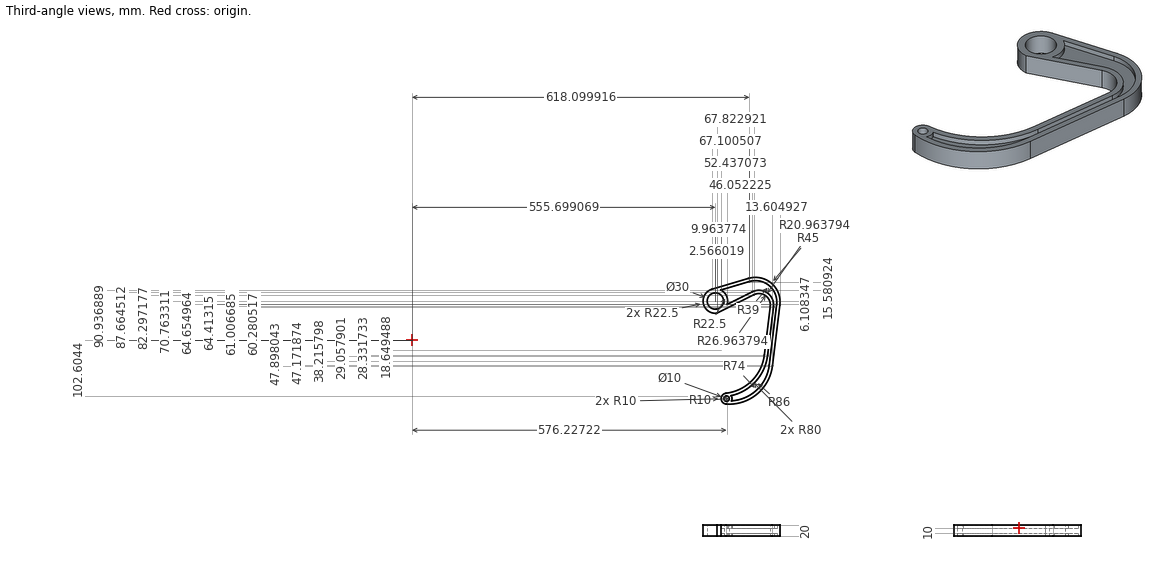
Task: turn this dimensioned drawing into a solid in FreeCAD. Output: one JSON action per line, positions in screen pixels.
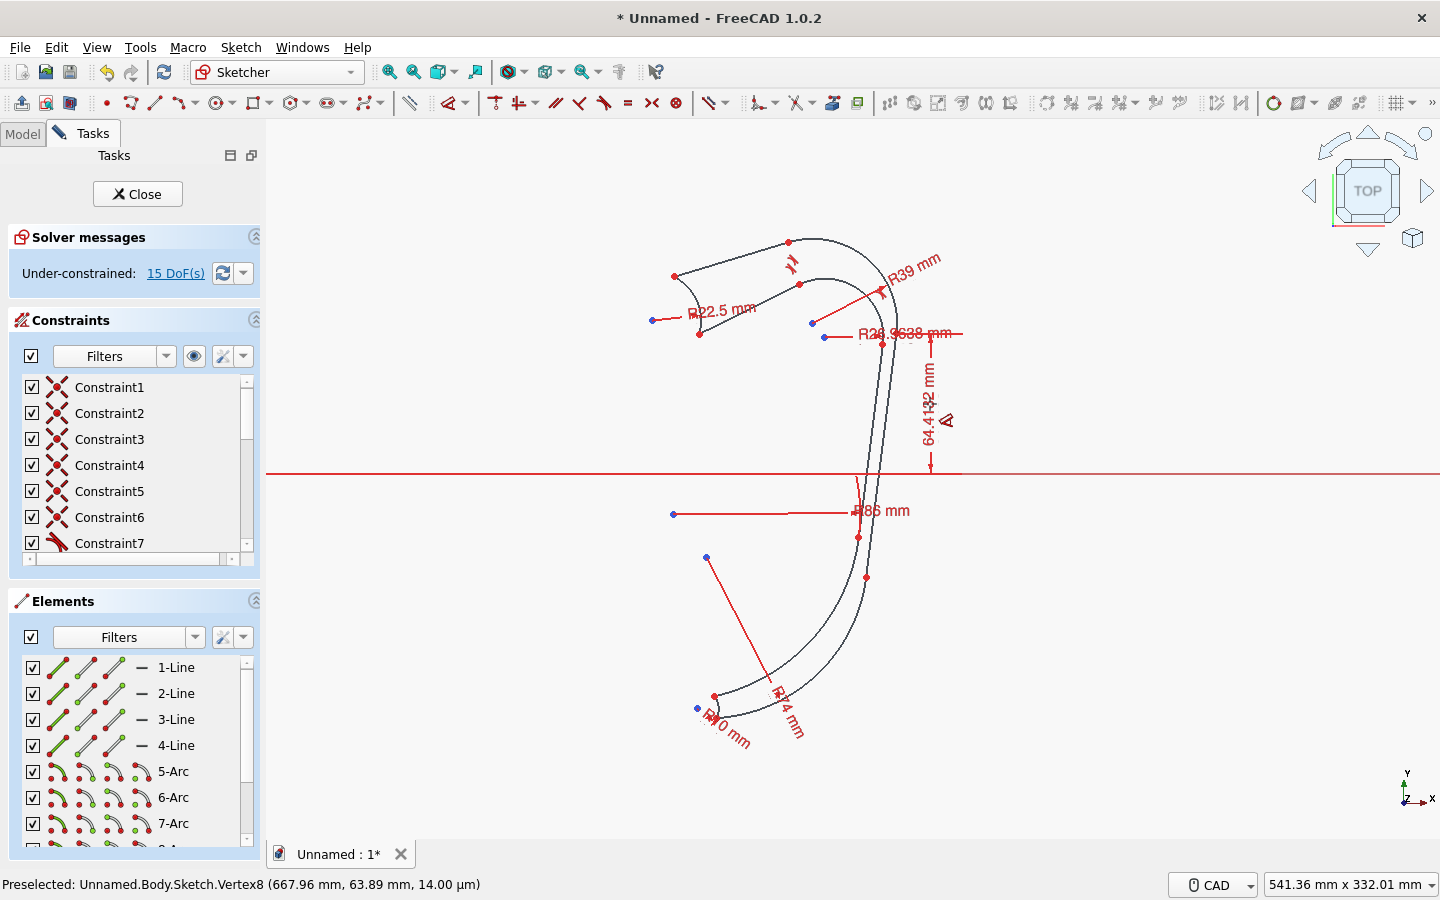
{"action": "left_click", "coordinate": [715, 696]}
{"action": "left_click", "coordinate": [749, 585]}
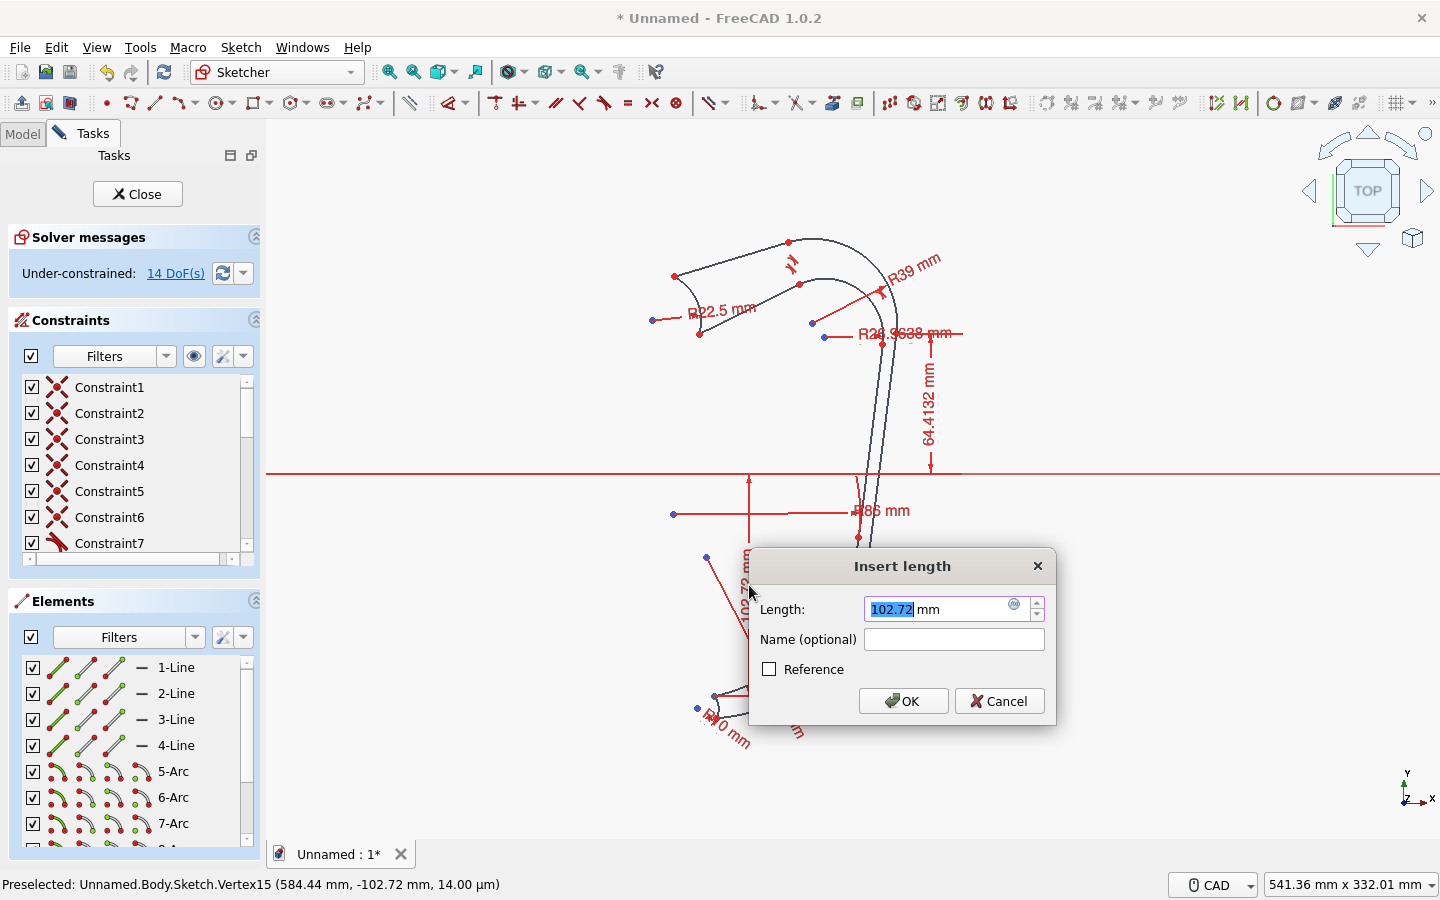
{"action": "type", "text": "102.6044"}
{"action": "key", "text": "Return"}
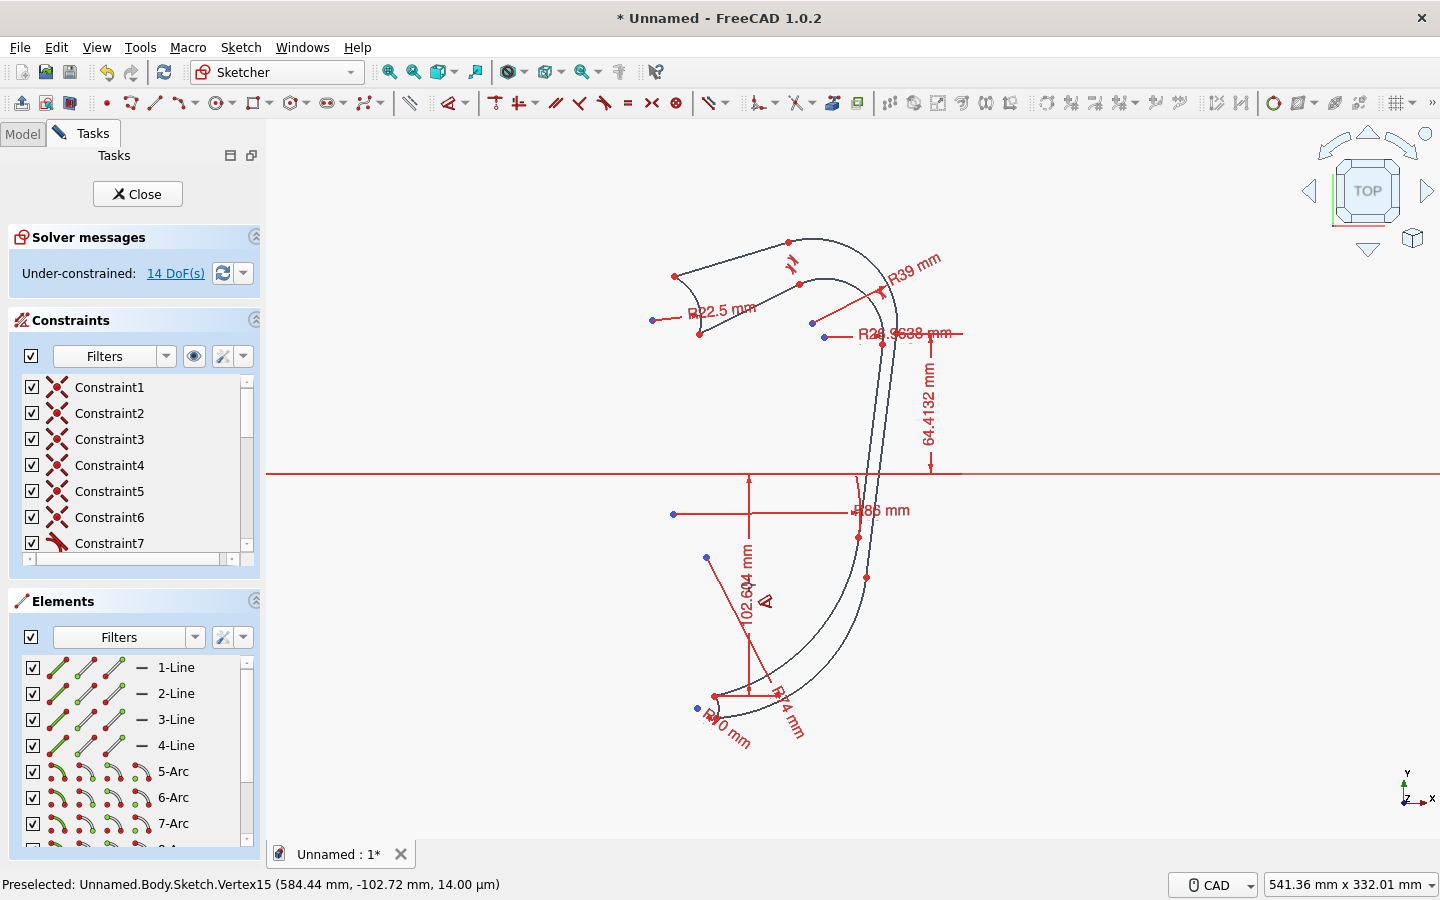
{"action": "left_click", "coordinate": [674, 277]}
{"action": "left_click", "coordinate": [708, 375]}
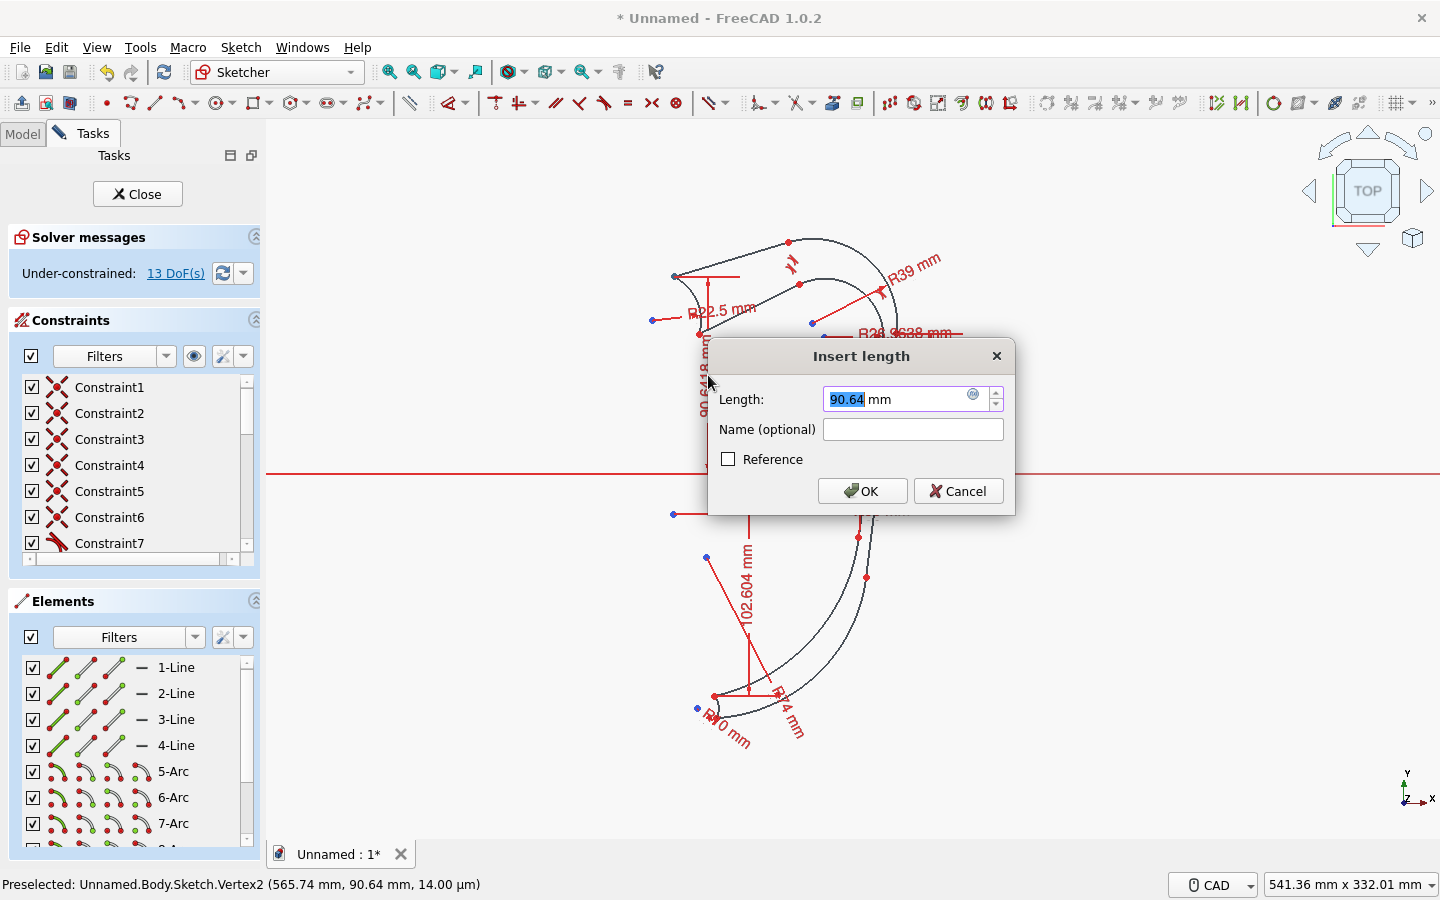
{"action": "type", "text": "90.936889"}
{"action": "key", "text": "Return"}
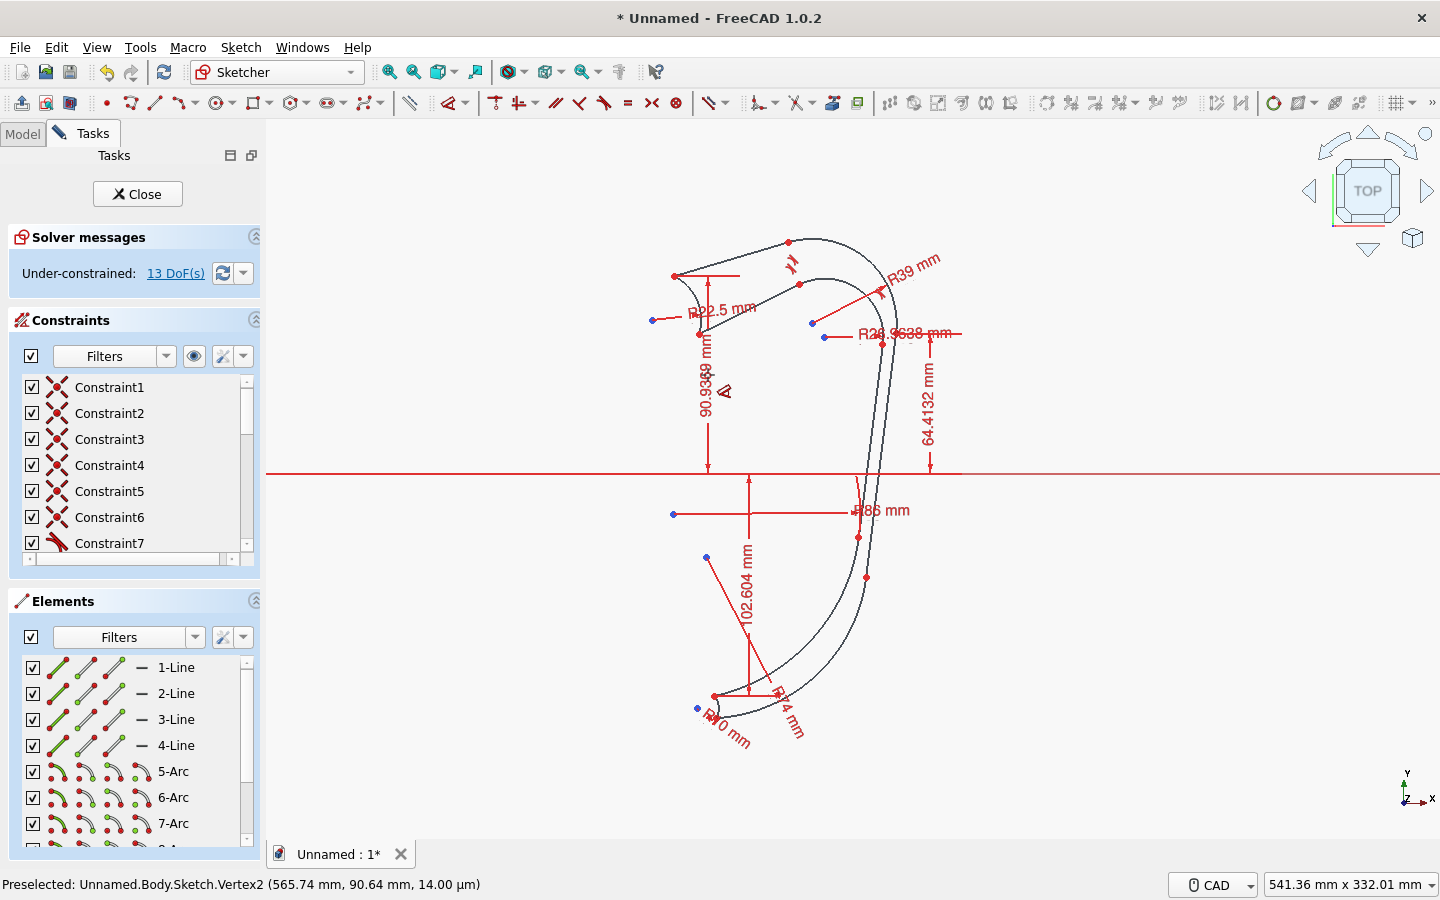
{"action": "left_click", "coordinate": [699, 334]}
{"action": "left_click", "coordinate": [733, 404]}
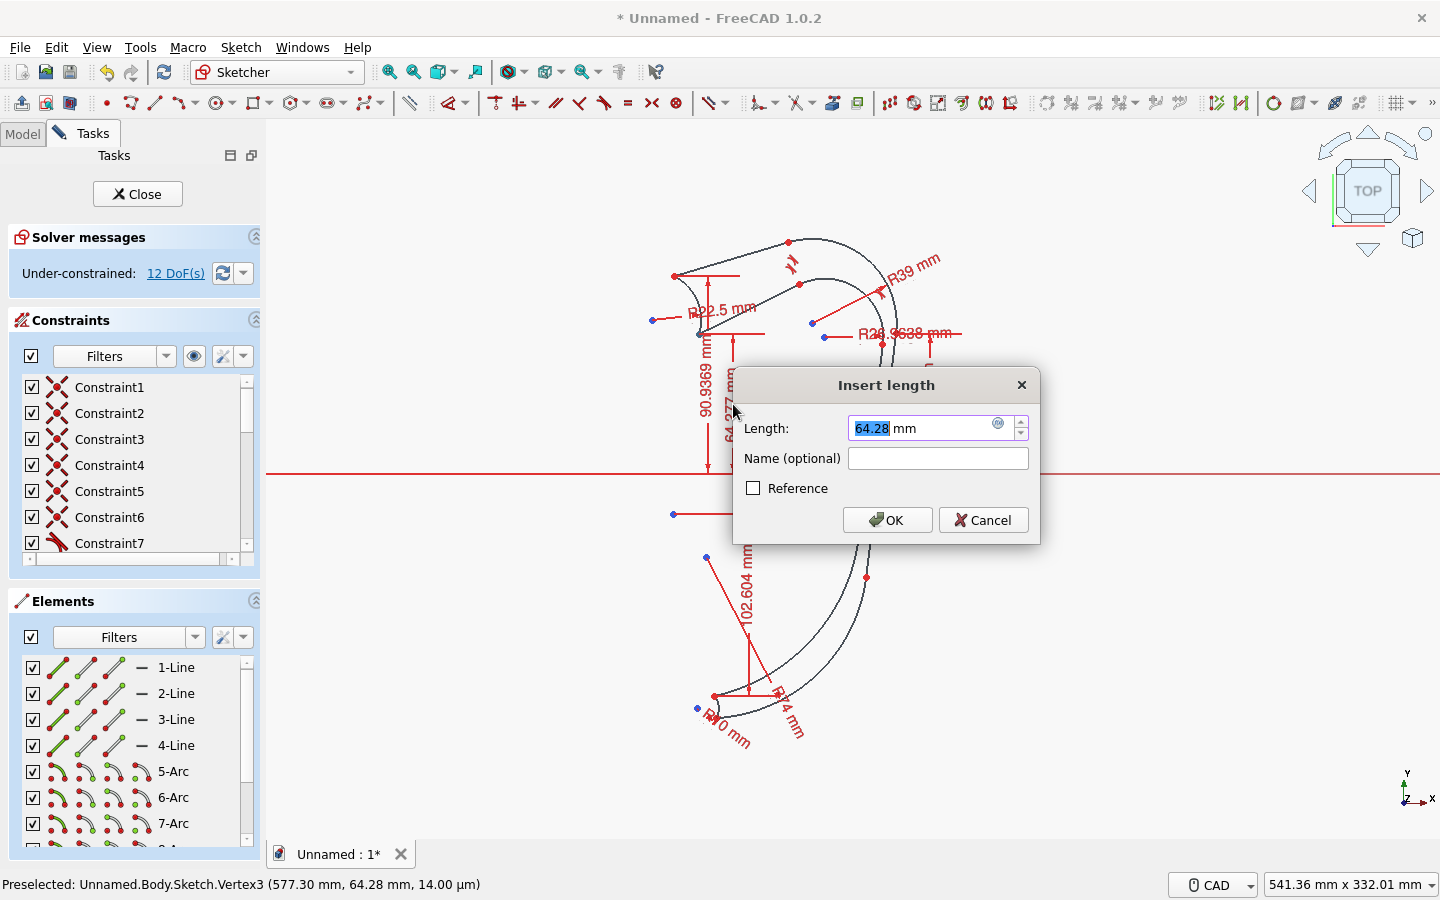
{"action": "type", "text": "64.654964"}
{"action": "key", "text": "Return"}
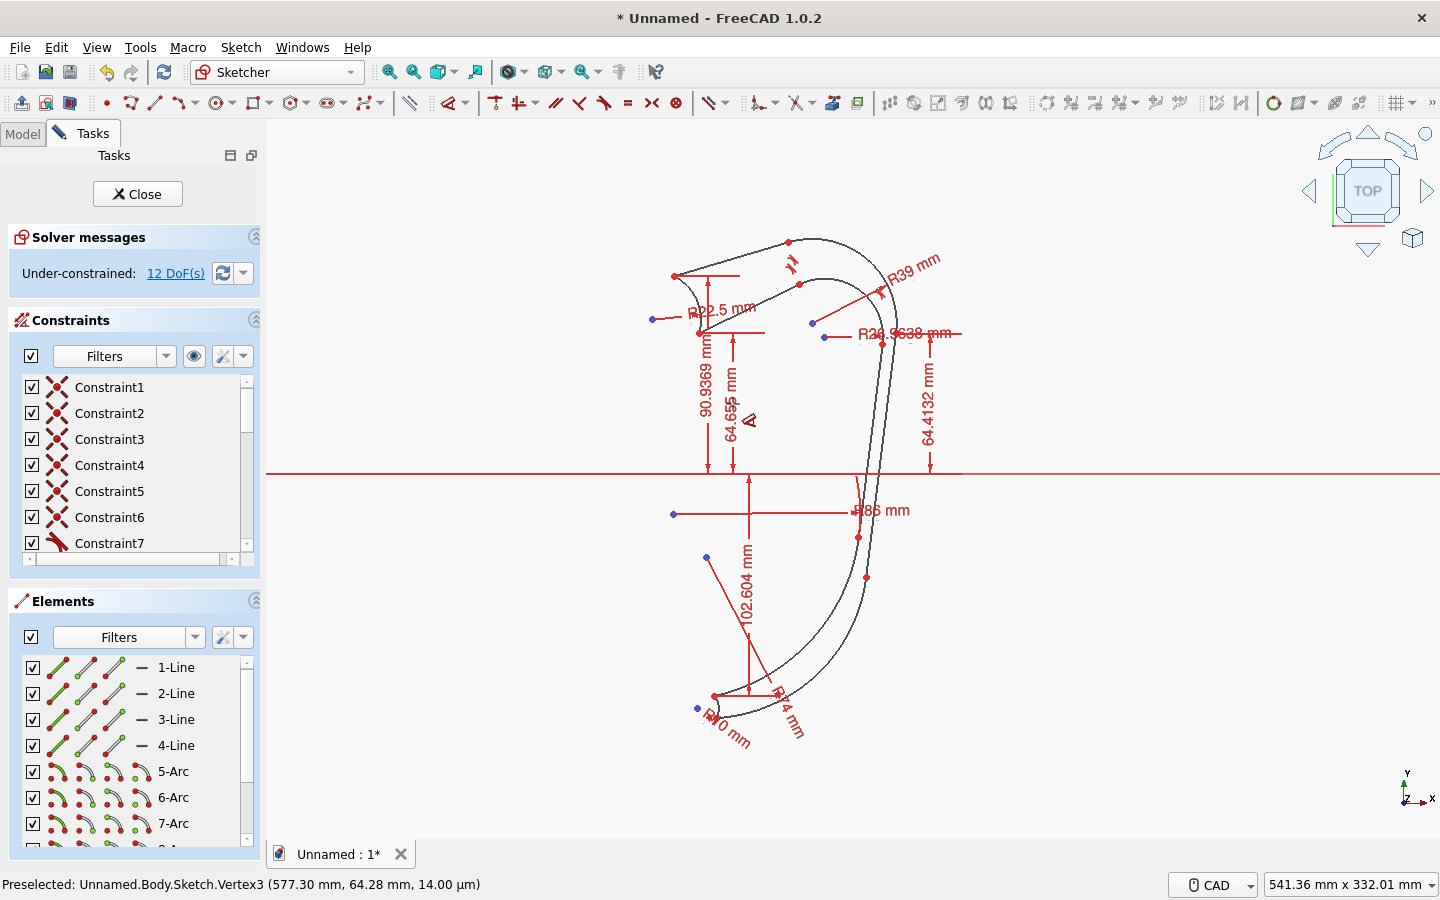
{"action": "left_click", "coordinate": [799, 285]}
{"action": "left_click", "coordinate": [833, 379]}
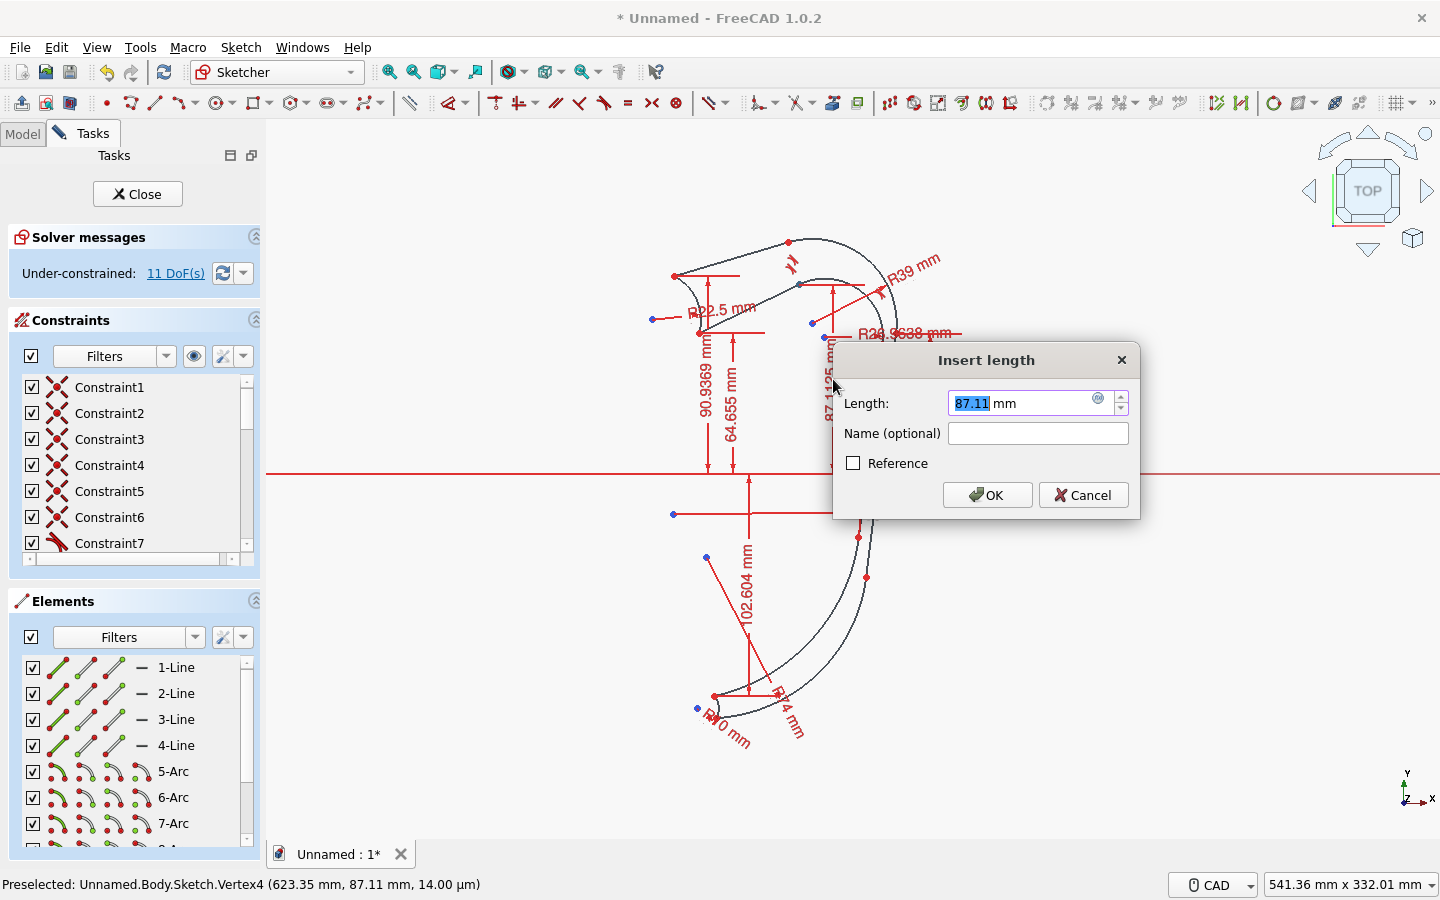
{"action": "type", "text": "87.664512"}
{"action": "key", "text": "Return"}